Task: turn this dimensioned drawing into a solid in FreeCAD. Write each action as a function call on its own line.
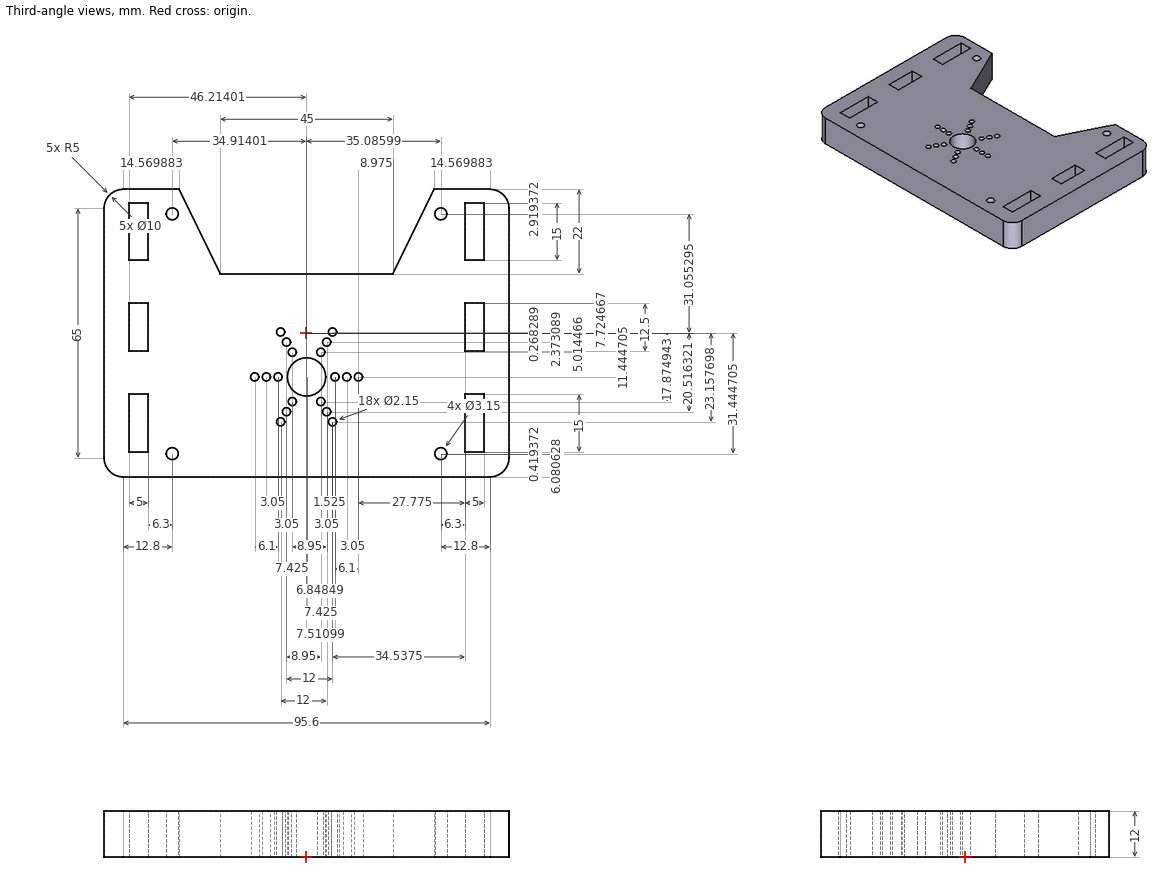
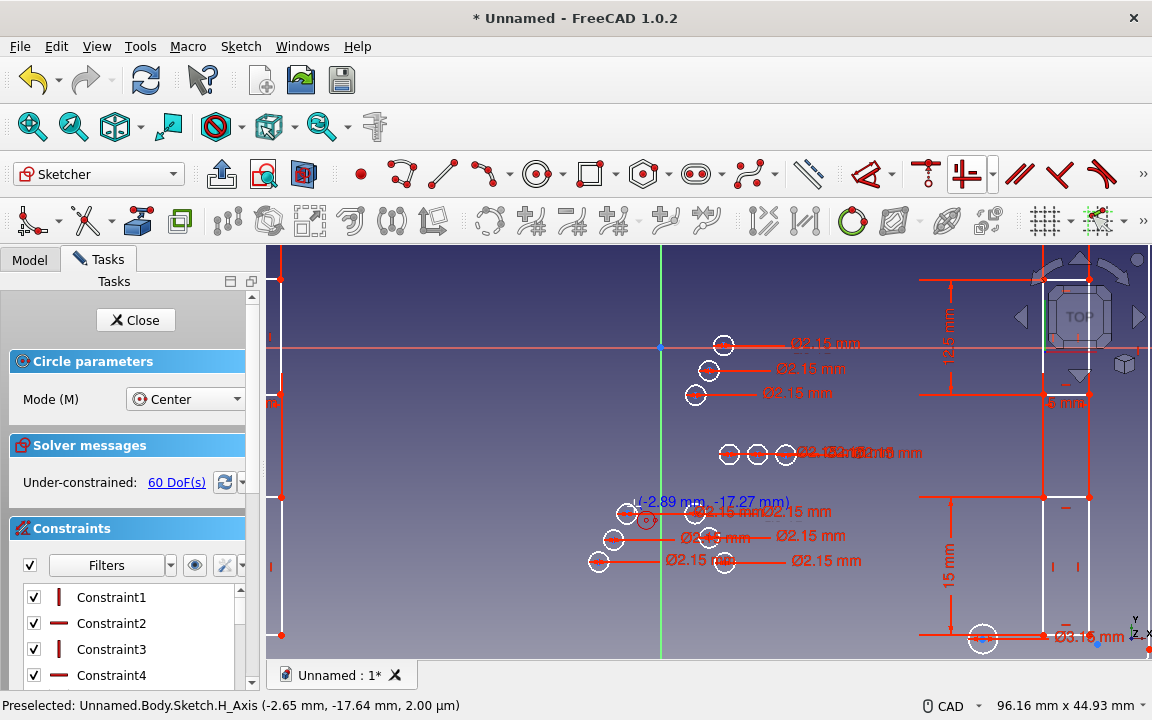
scroll(628, 512, down, 5)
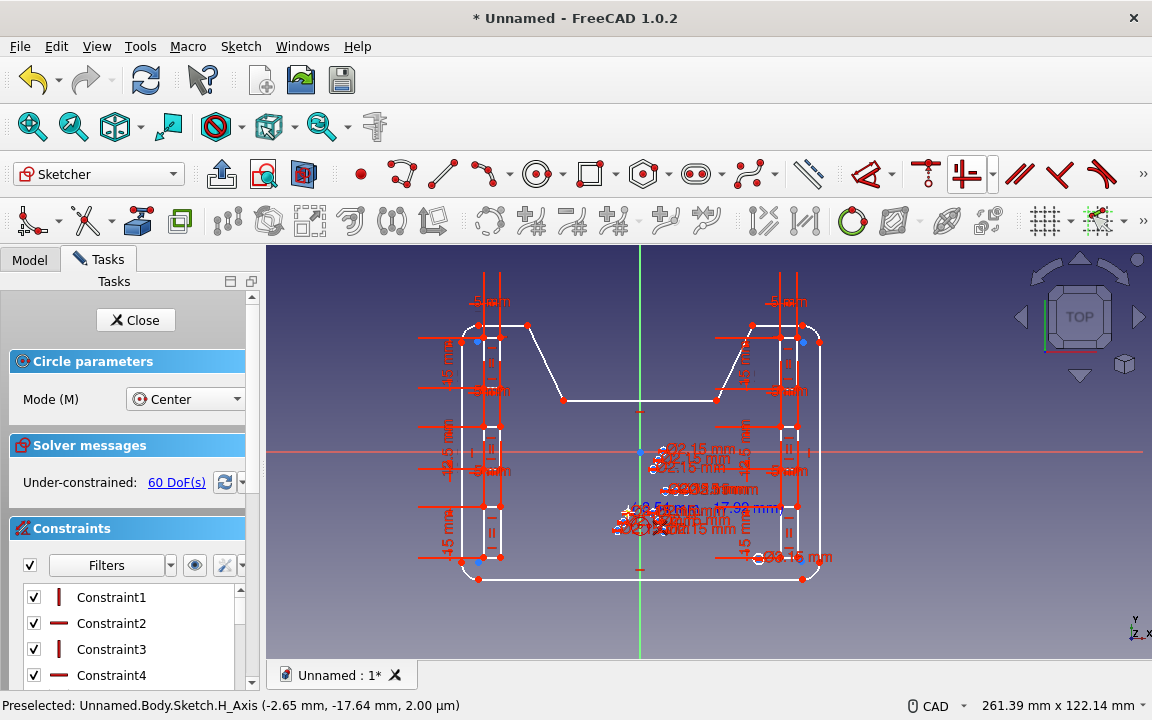
scroll(522, 559, up, 8)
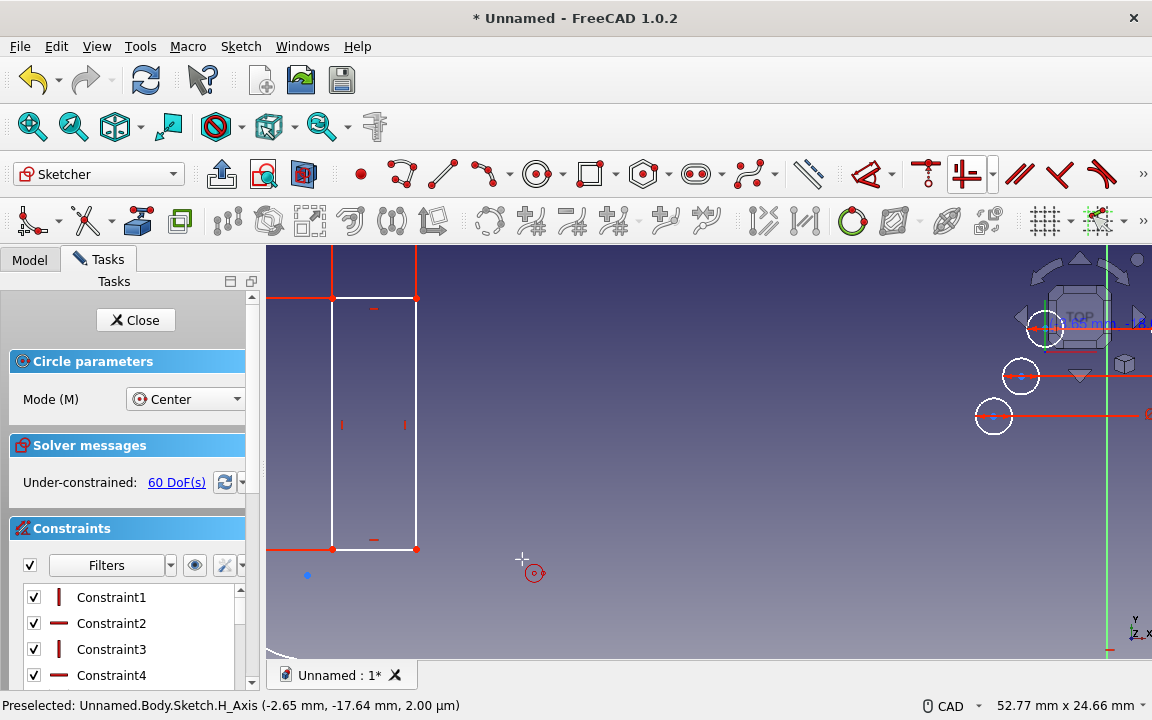
scroll(522, 560, down, 8)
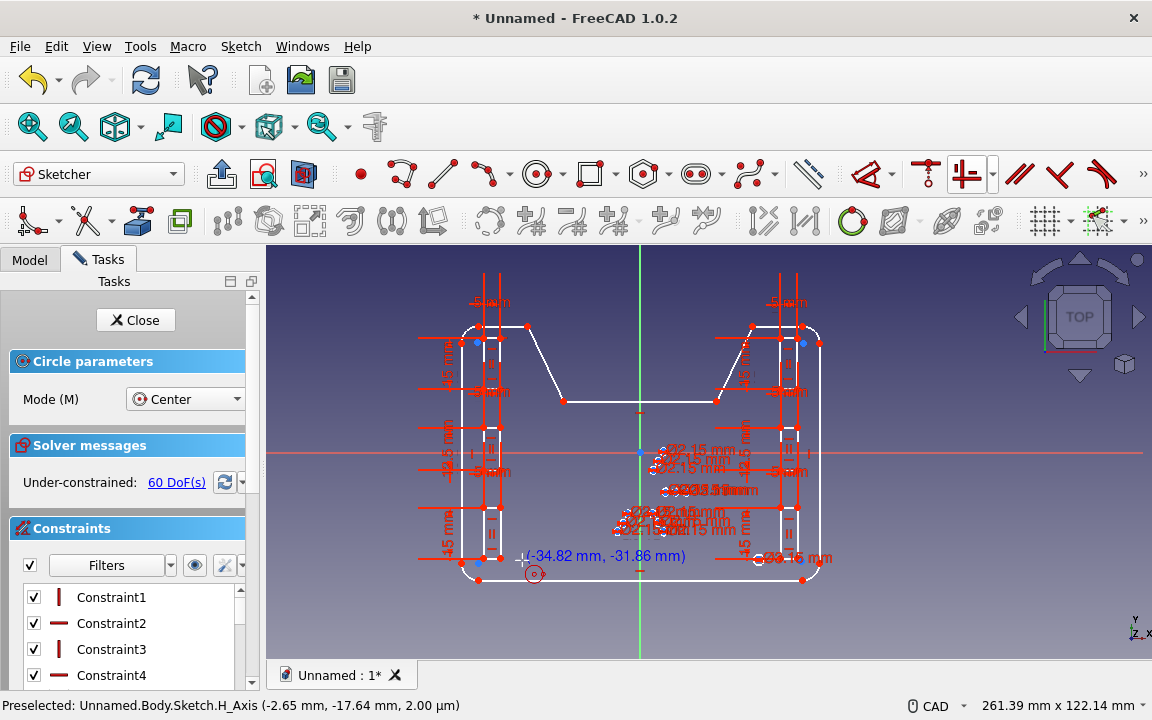
click(522, 559)
move(526, 556)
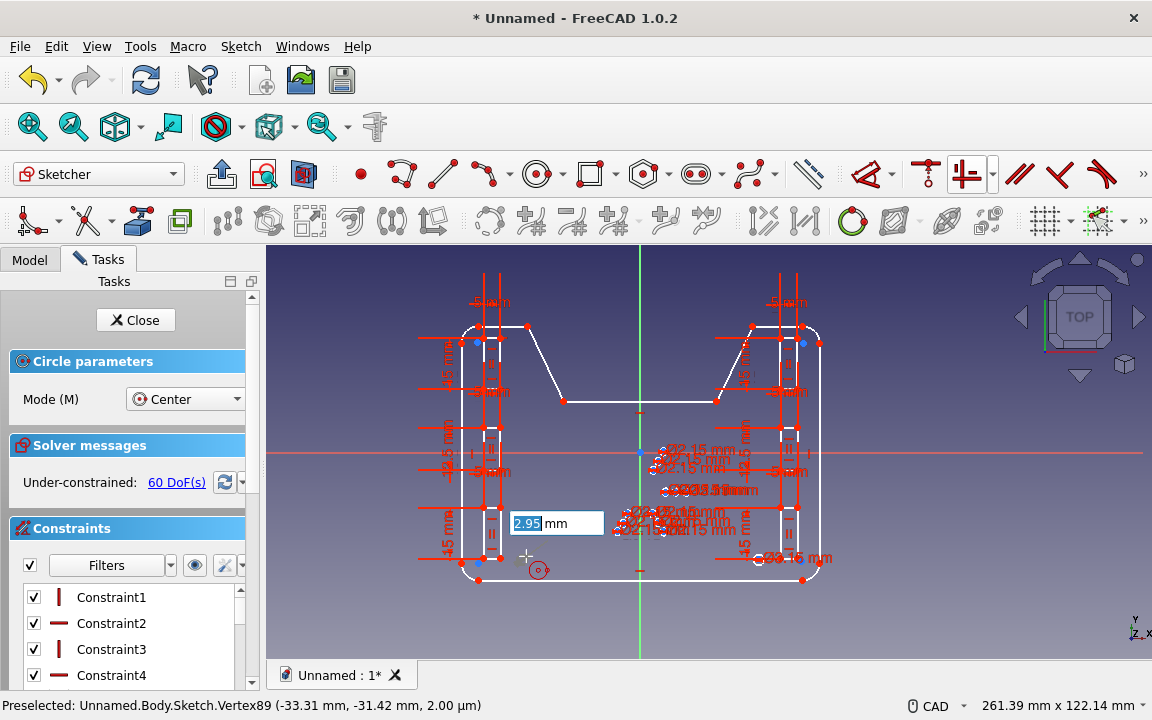
text(3.15)
key(Return)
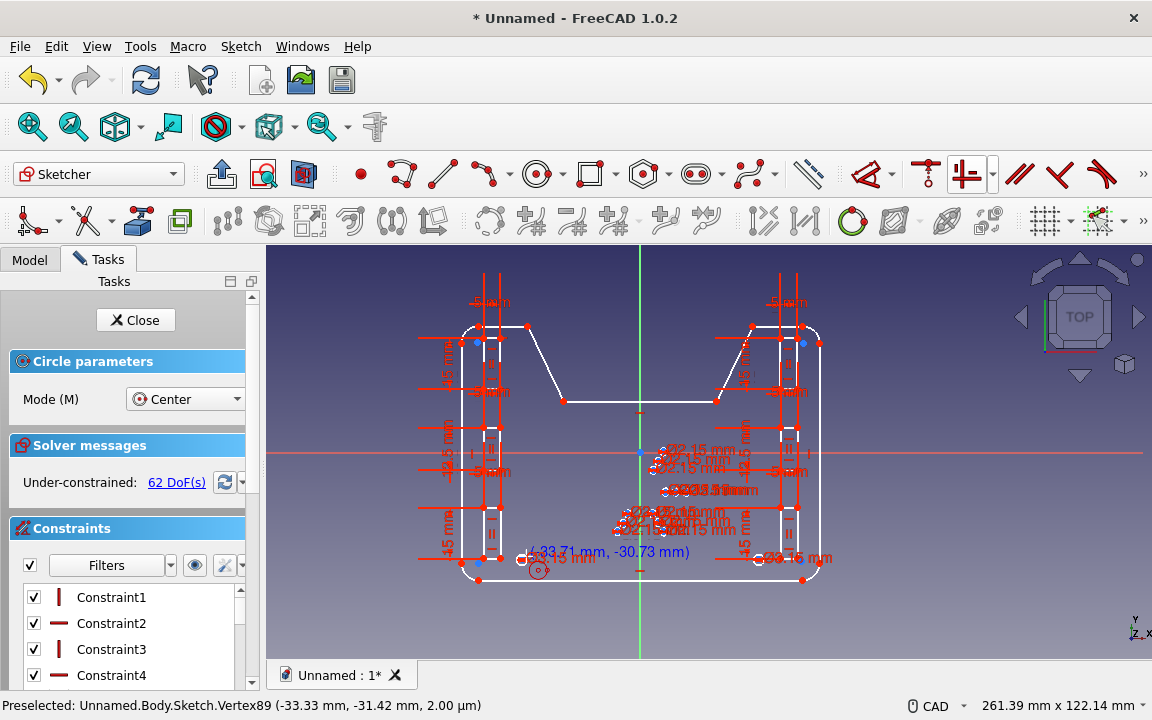
scroll(641, 492, up, 20)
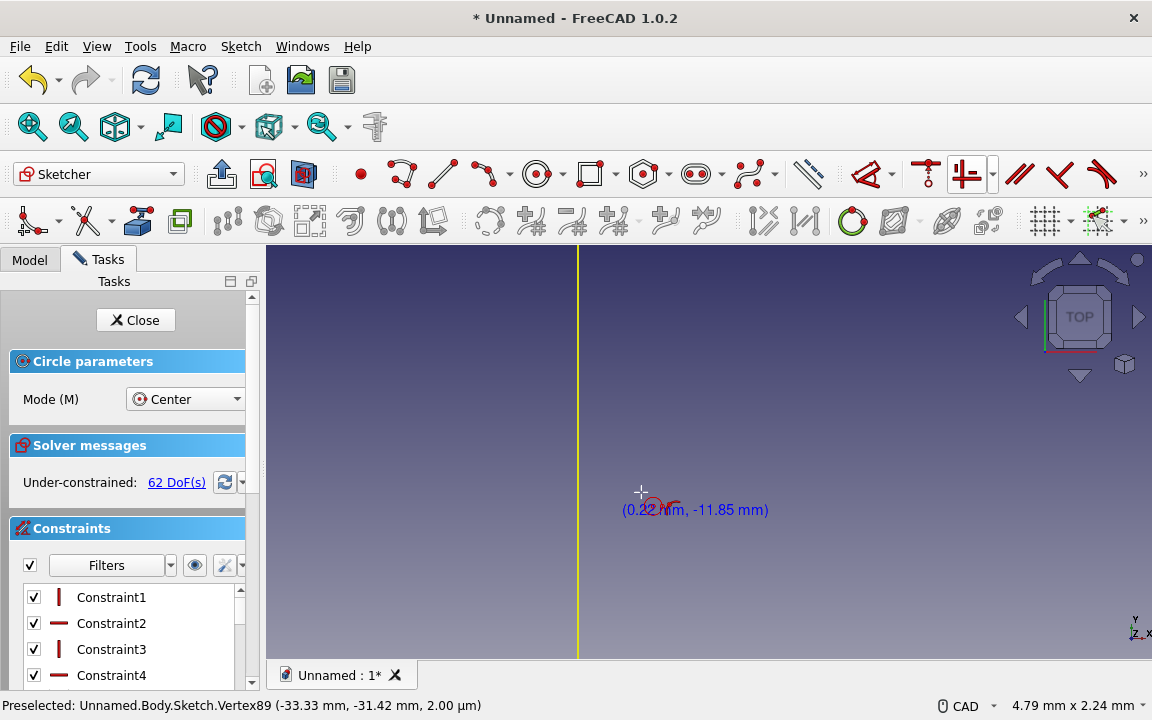
click(594, 439)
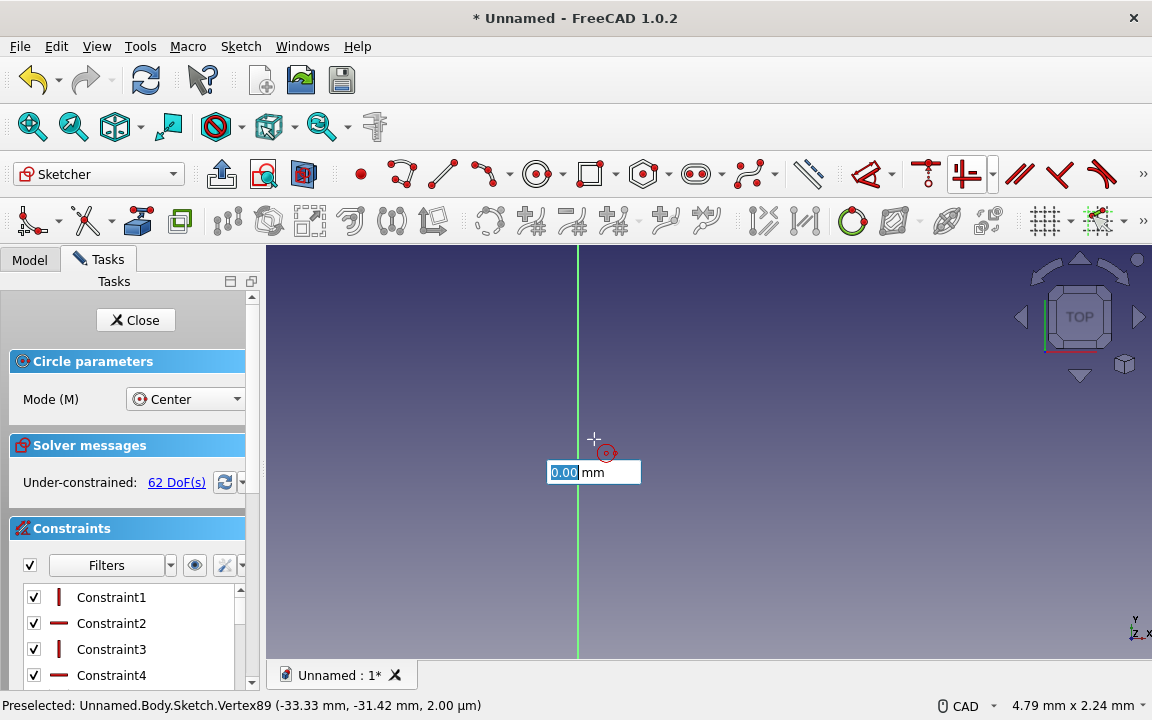
scroll(640, 452, down, 15)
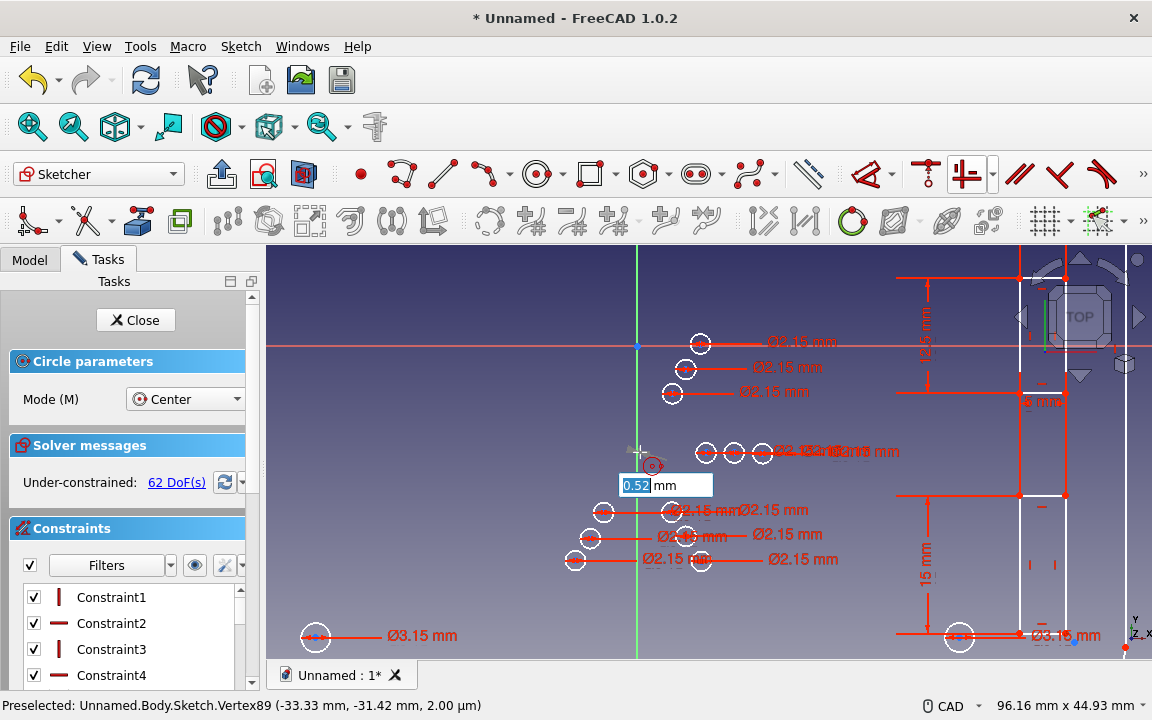
scroll(642, 513, down, 5)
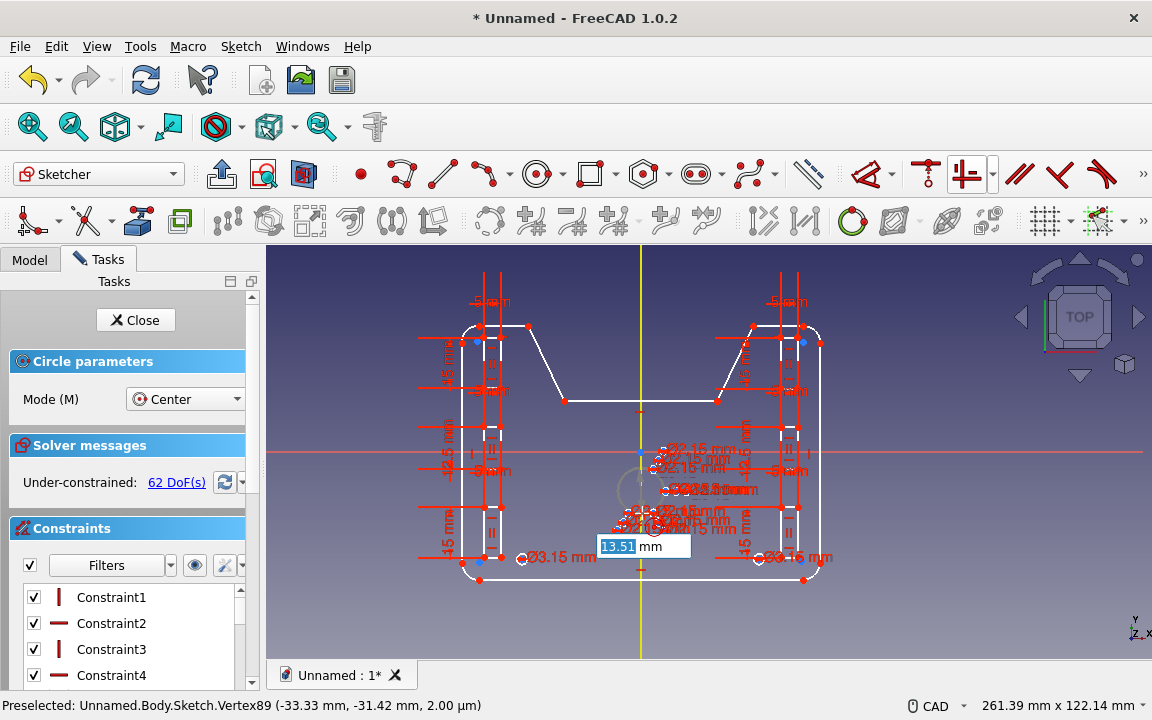
scroll(653, 479, up, 5)
move(652, 478)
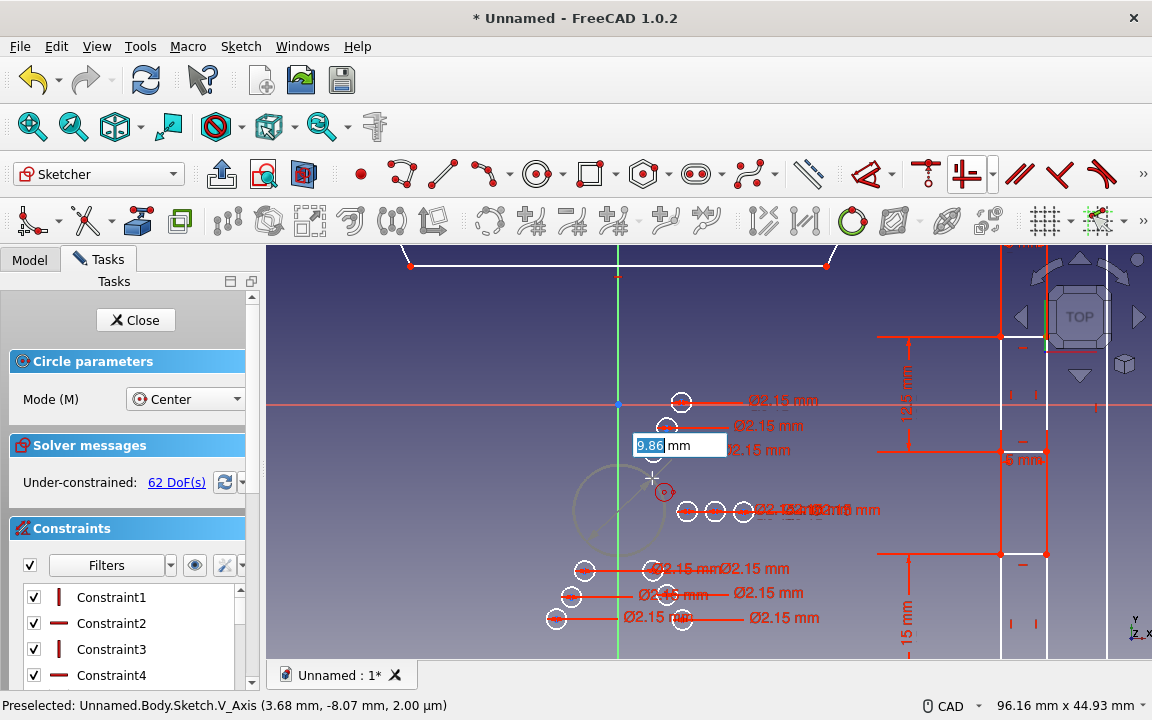
text(10)
key(Return)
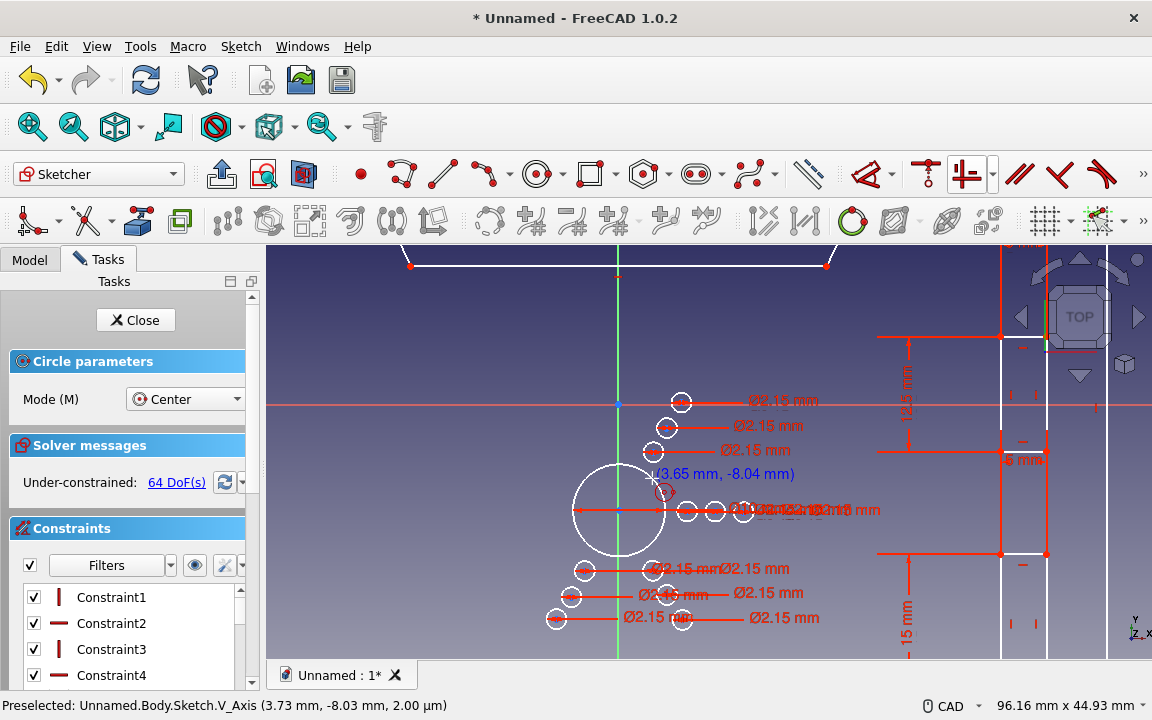
scroll(551, 510, up, 5)